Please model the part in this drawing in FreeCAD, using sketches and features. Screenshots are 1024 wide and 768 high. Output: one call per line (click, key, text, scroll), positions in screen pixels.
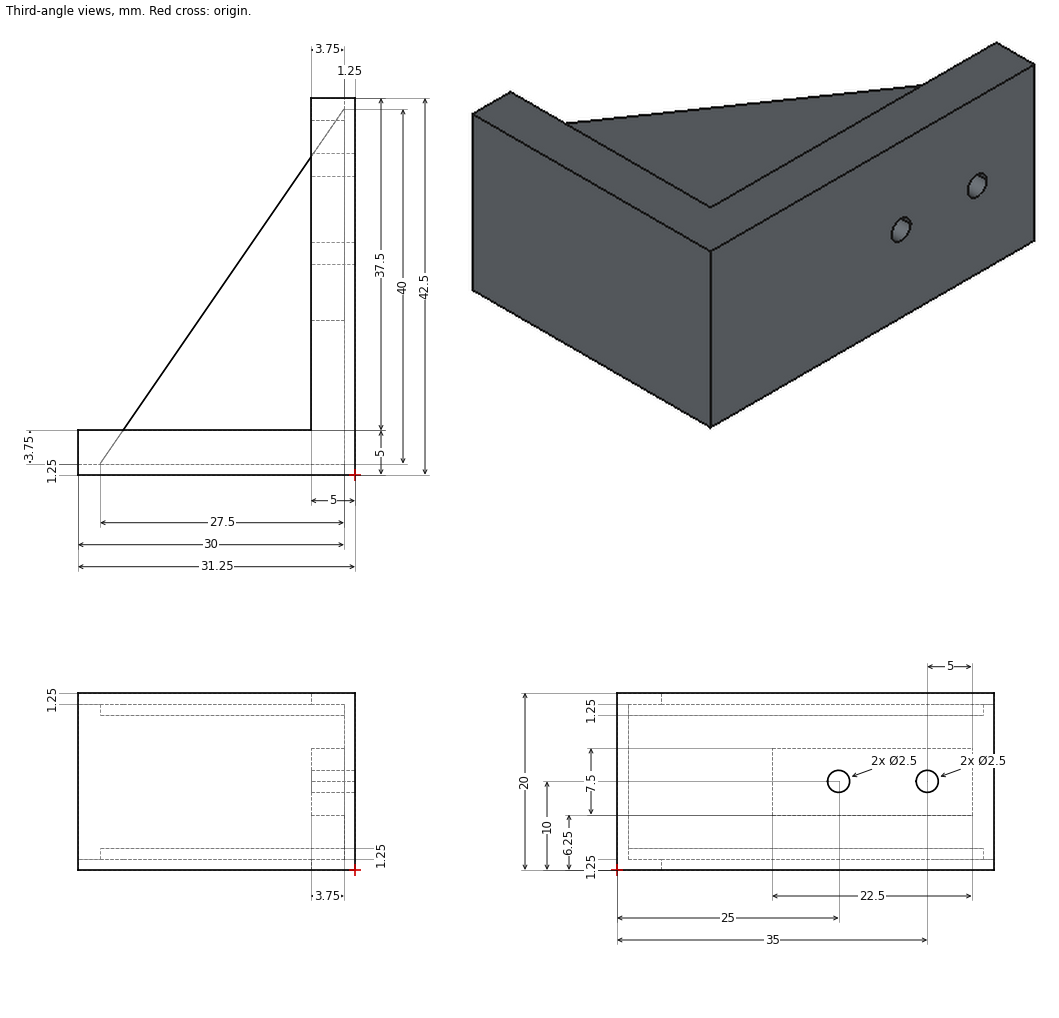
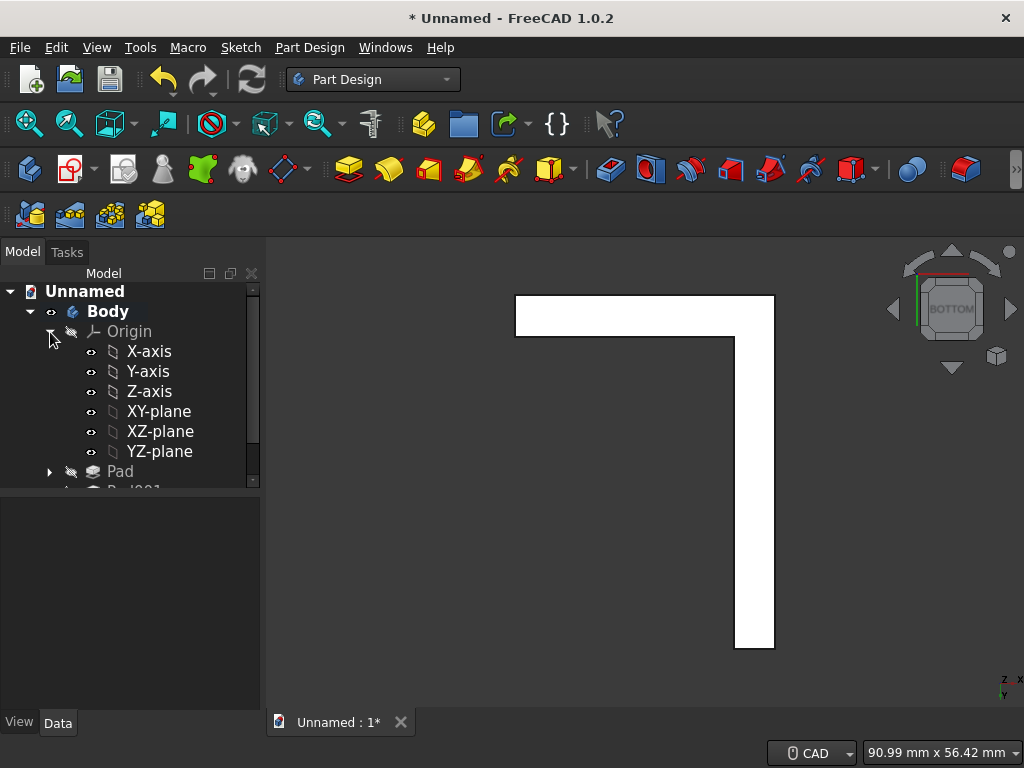
click(136, 412)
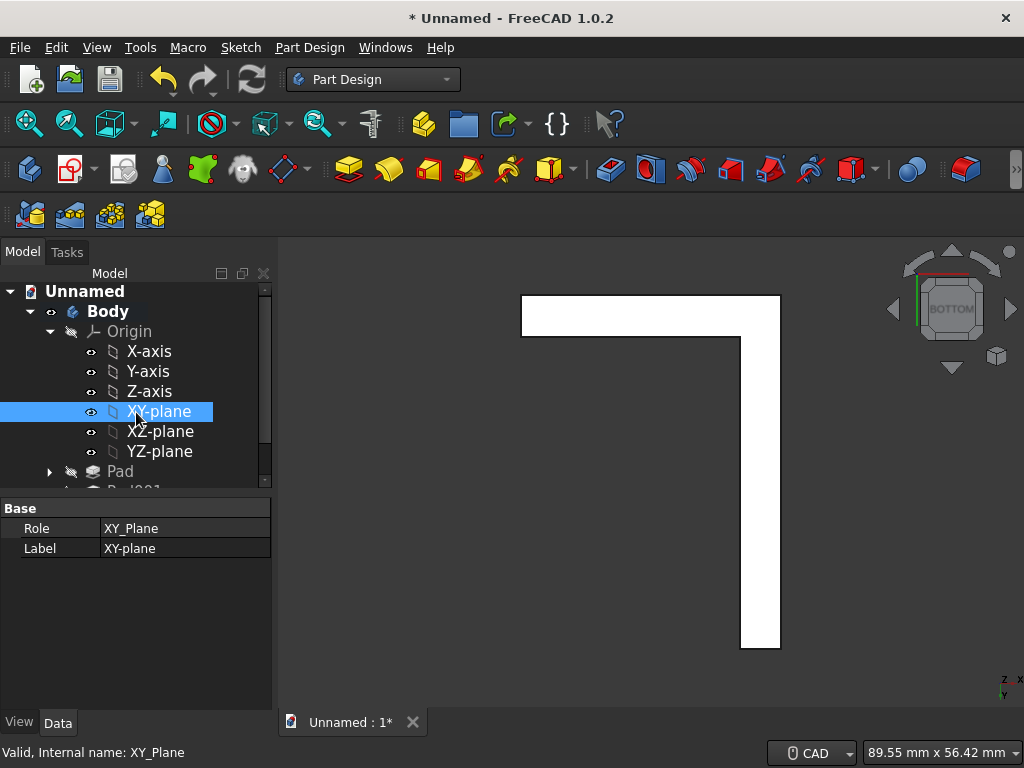
click(284, 170)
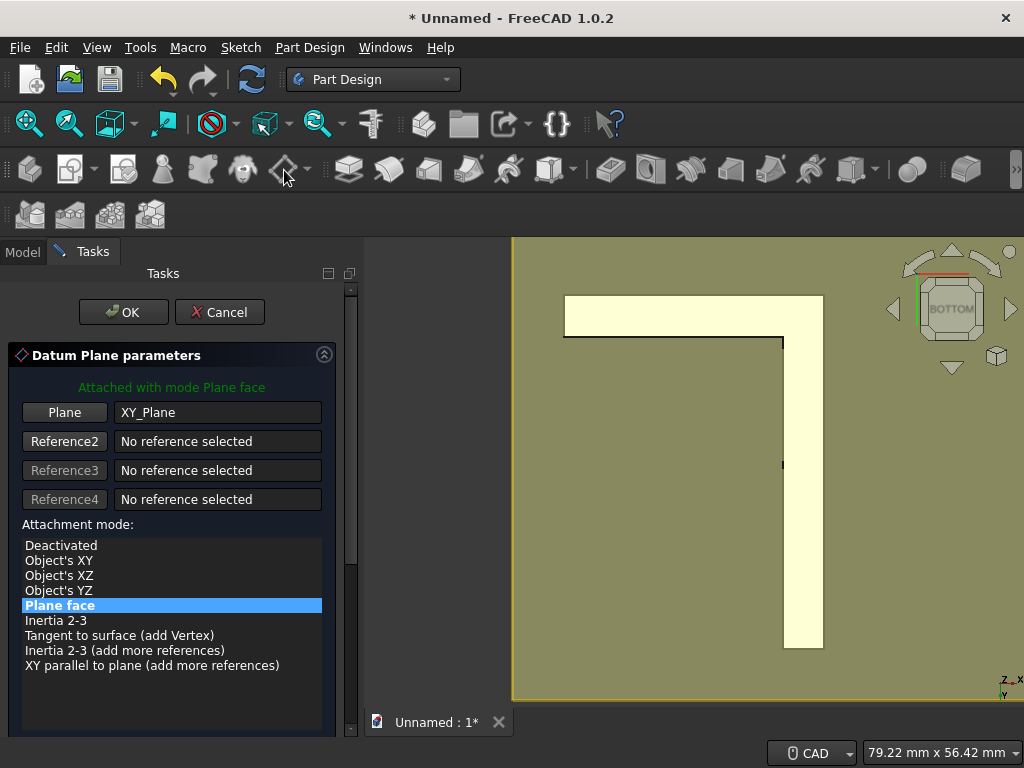
scroll(351, 510, down, 3)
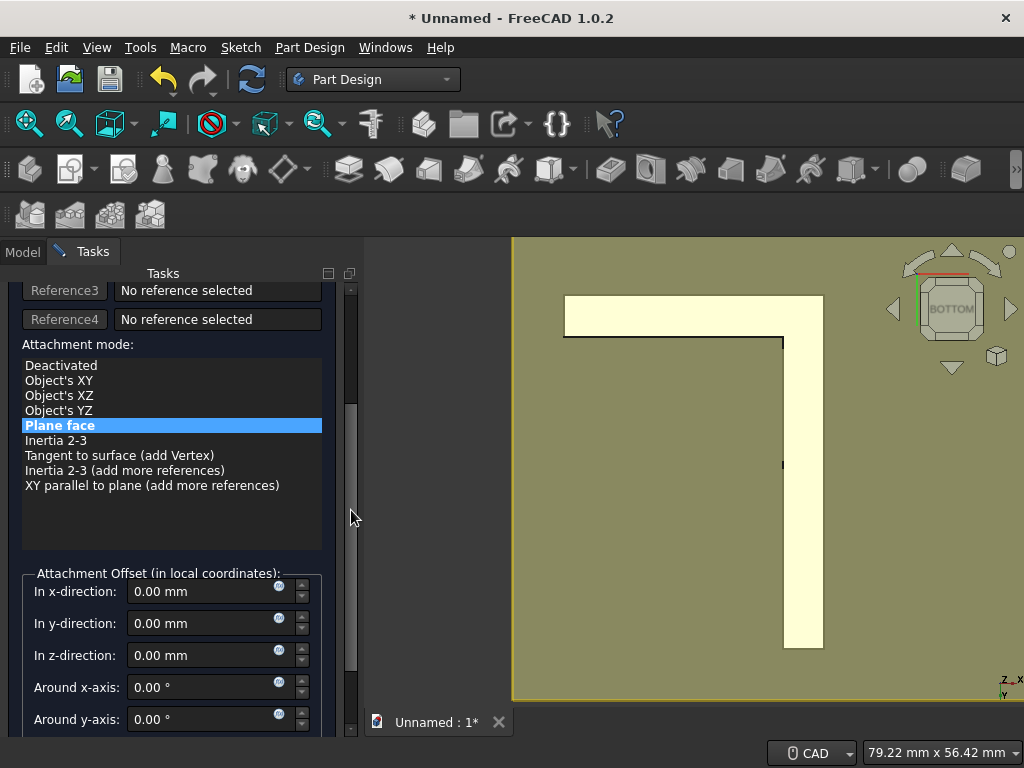
triple_click(210, 655)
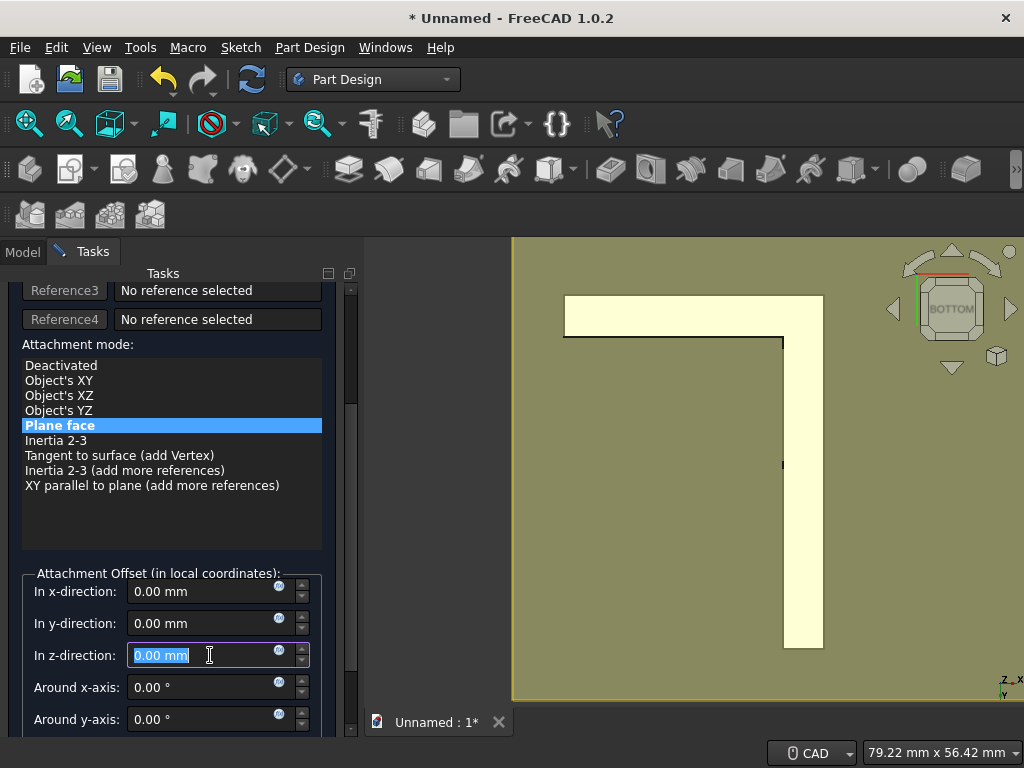
text(1.25)
key(Tab)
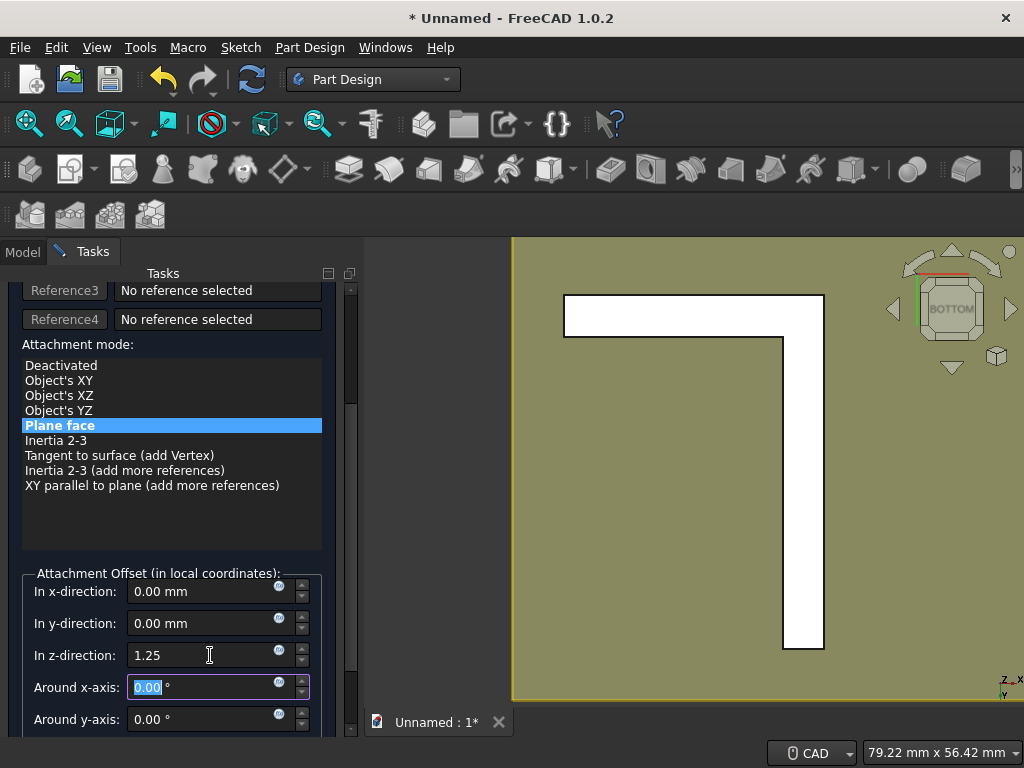
scroll(351, 510, up, 4)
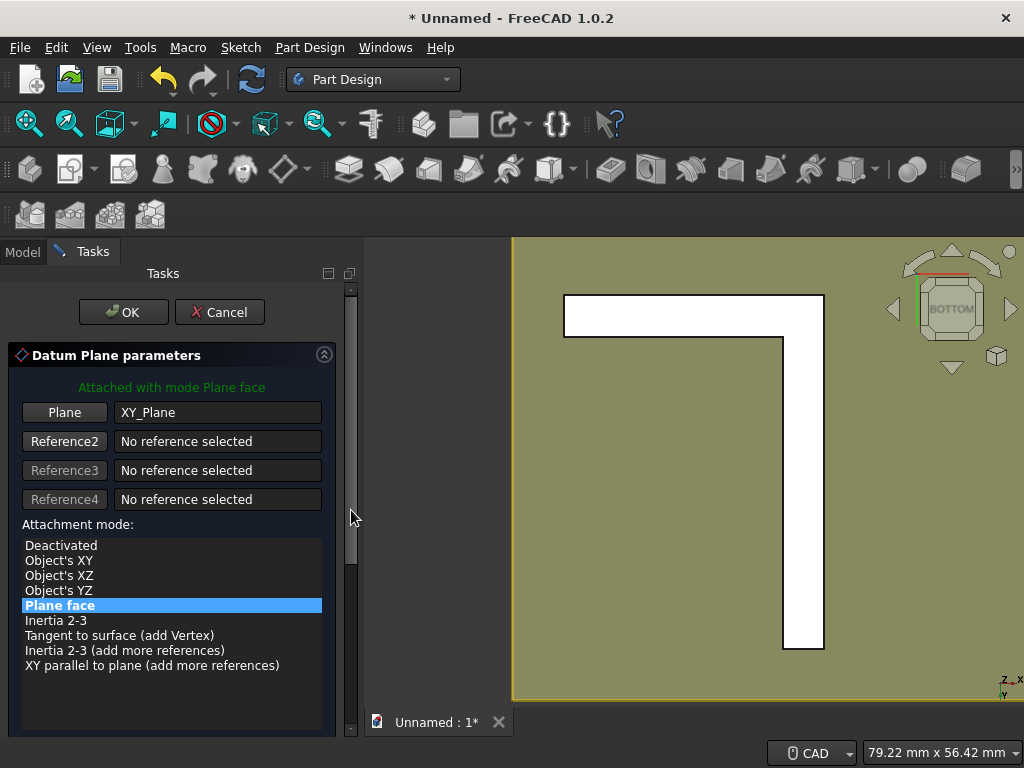
click(124, 312)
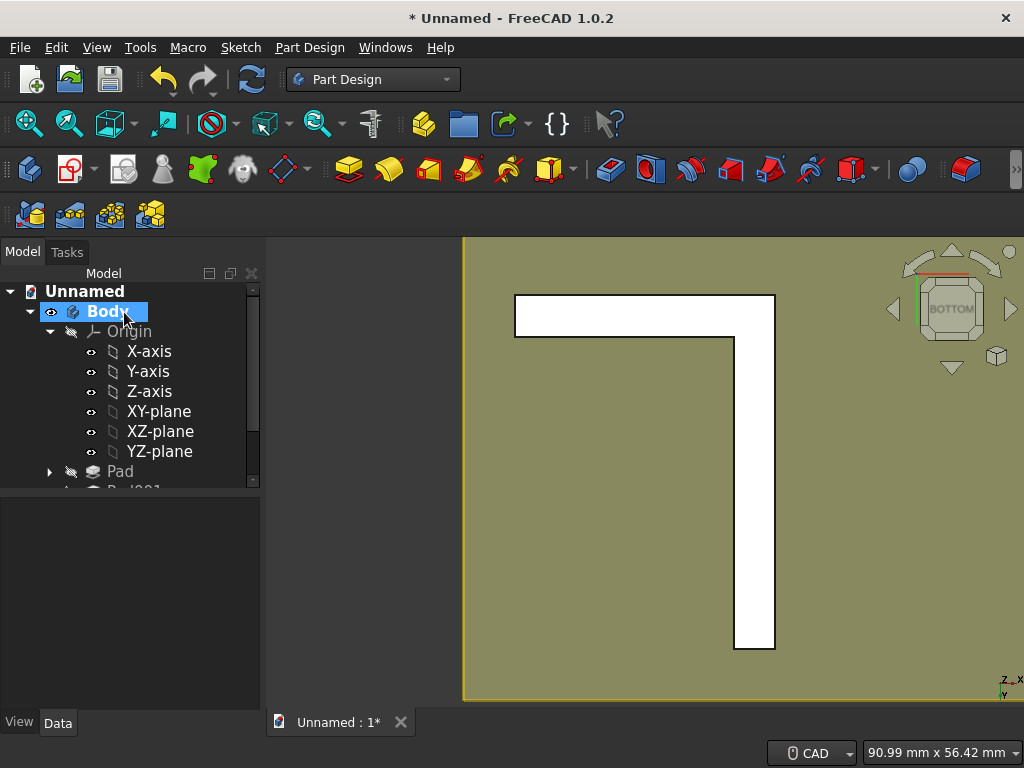
scroll(100, 387, down, 3)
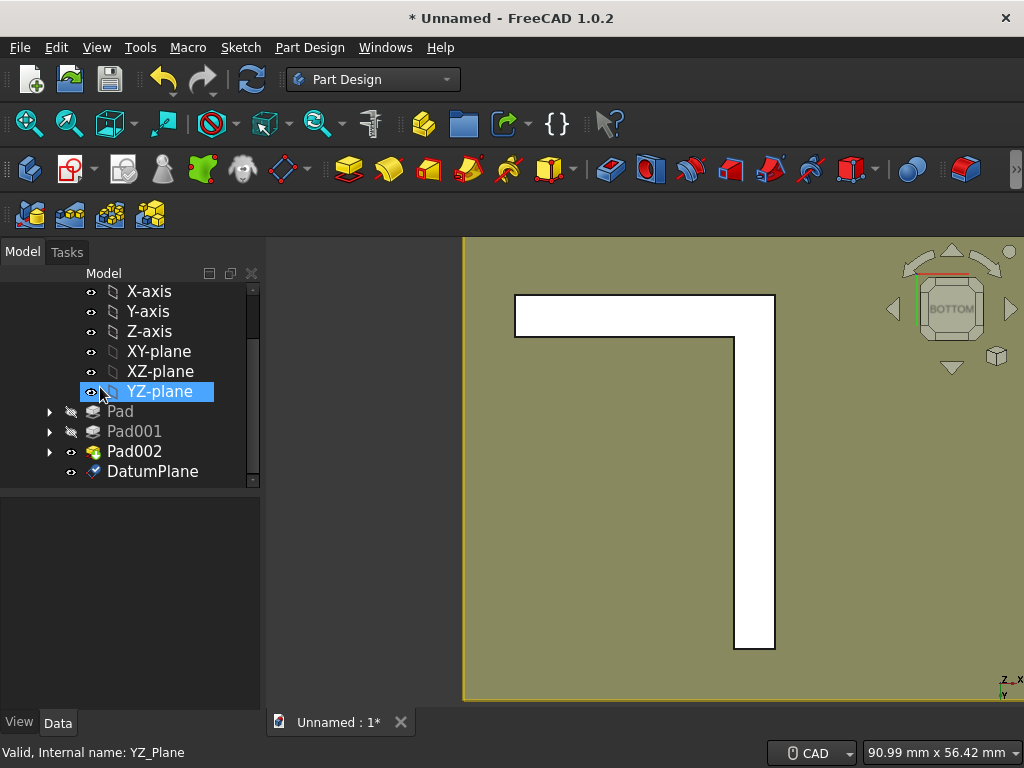
click(116, 472)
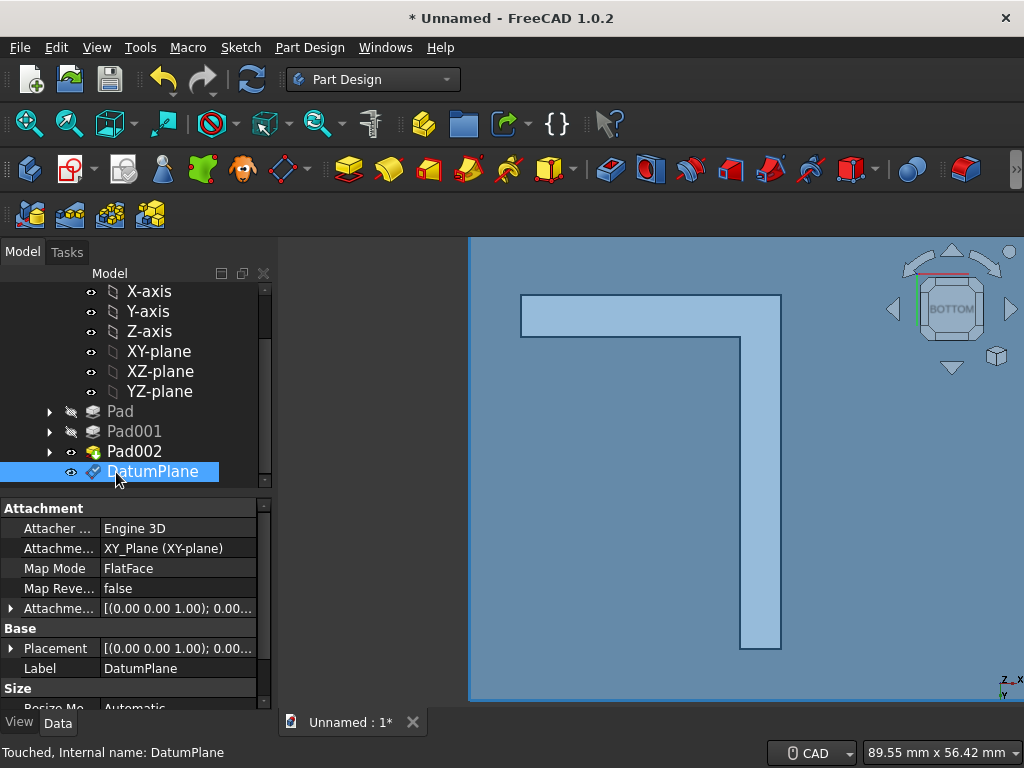
click(70, 170)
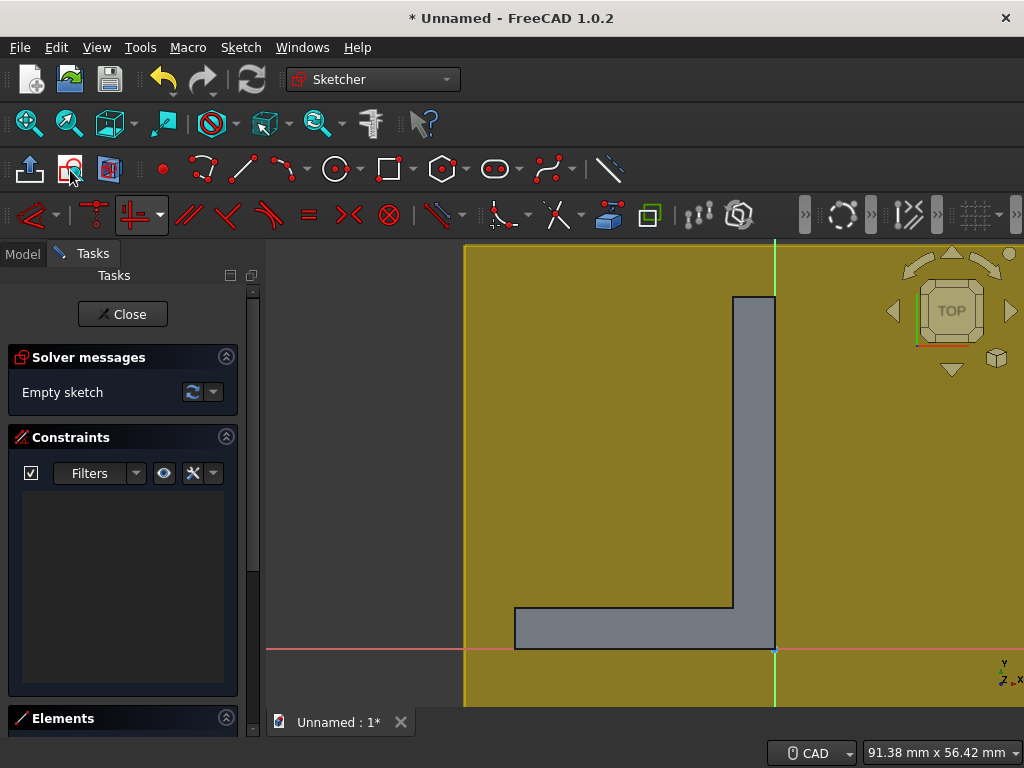
click(110, 170)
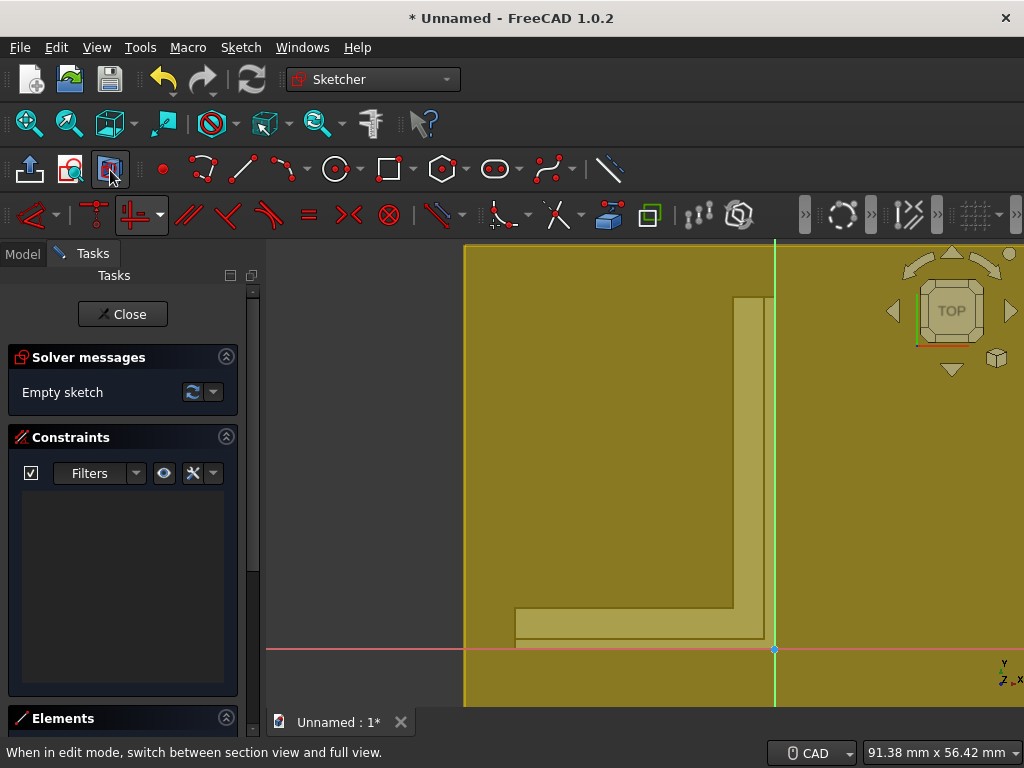
key(g)
key(m)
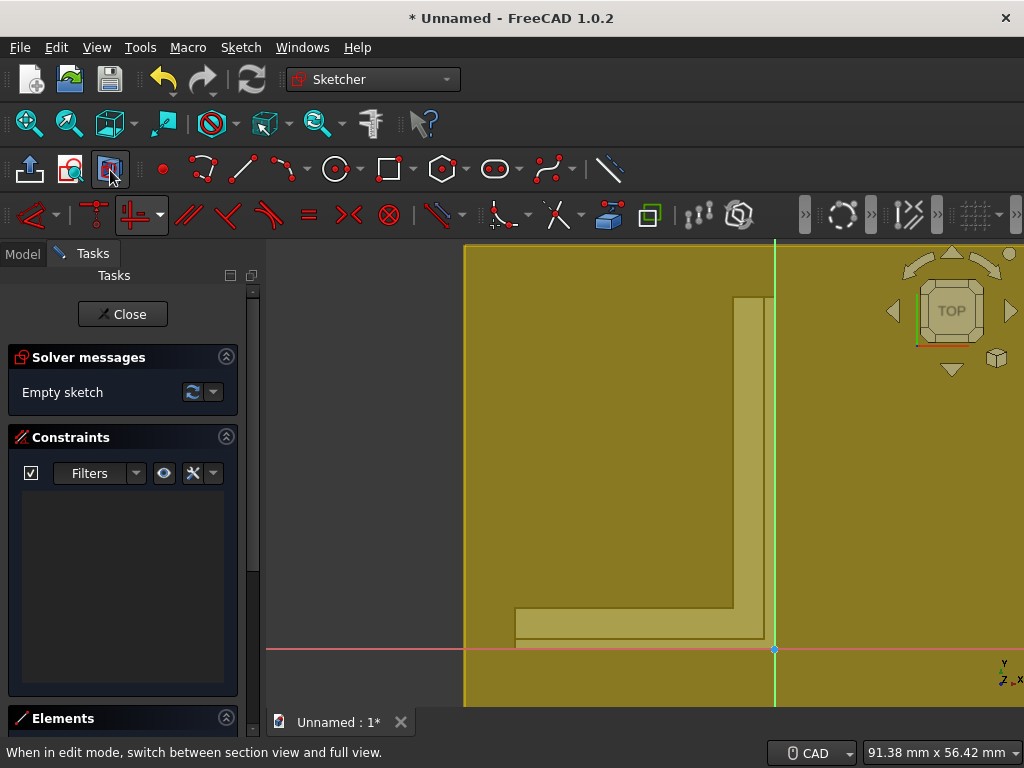
scroll(764, 639, up, 3)